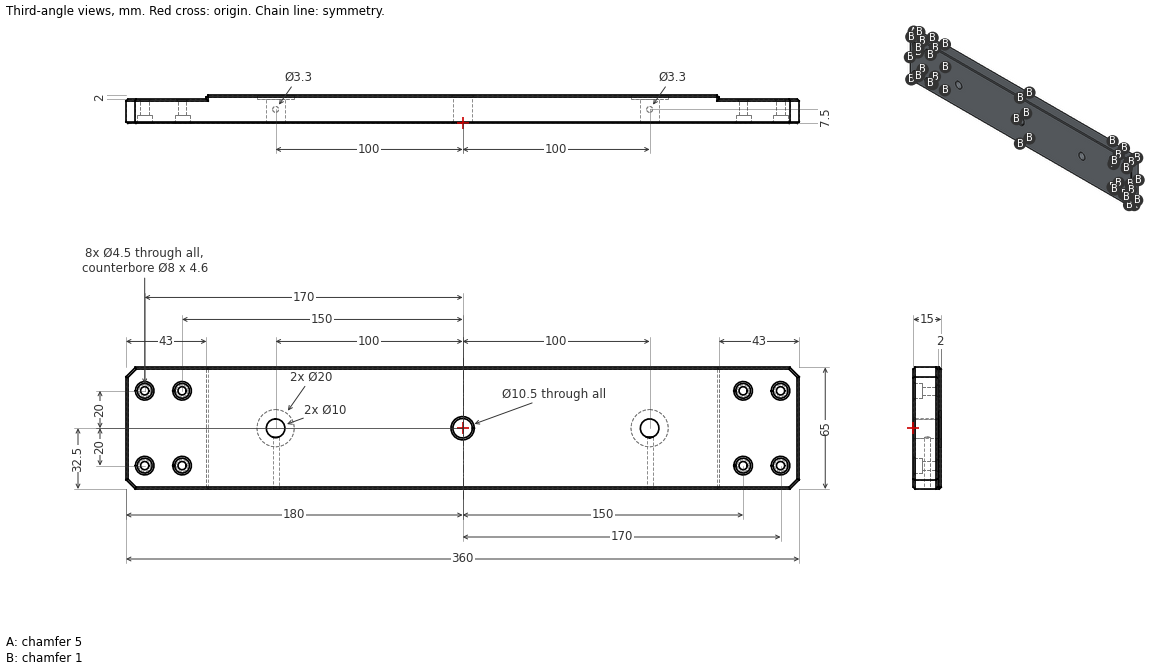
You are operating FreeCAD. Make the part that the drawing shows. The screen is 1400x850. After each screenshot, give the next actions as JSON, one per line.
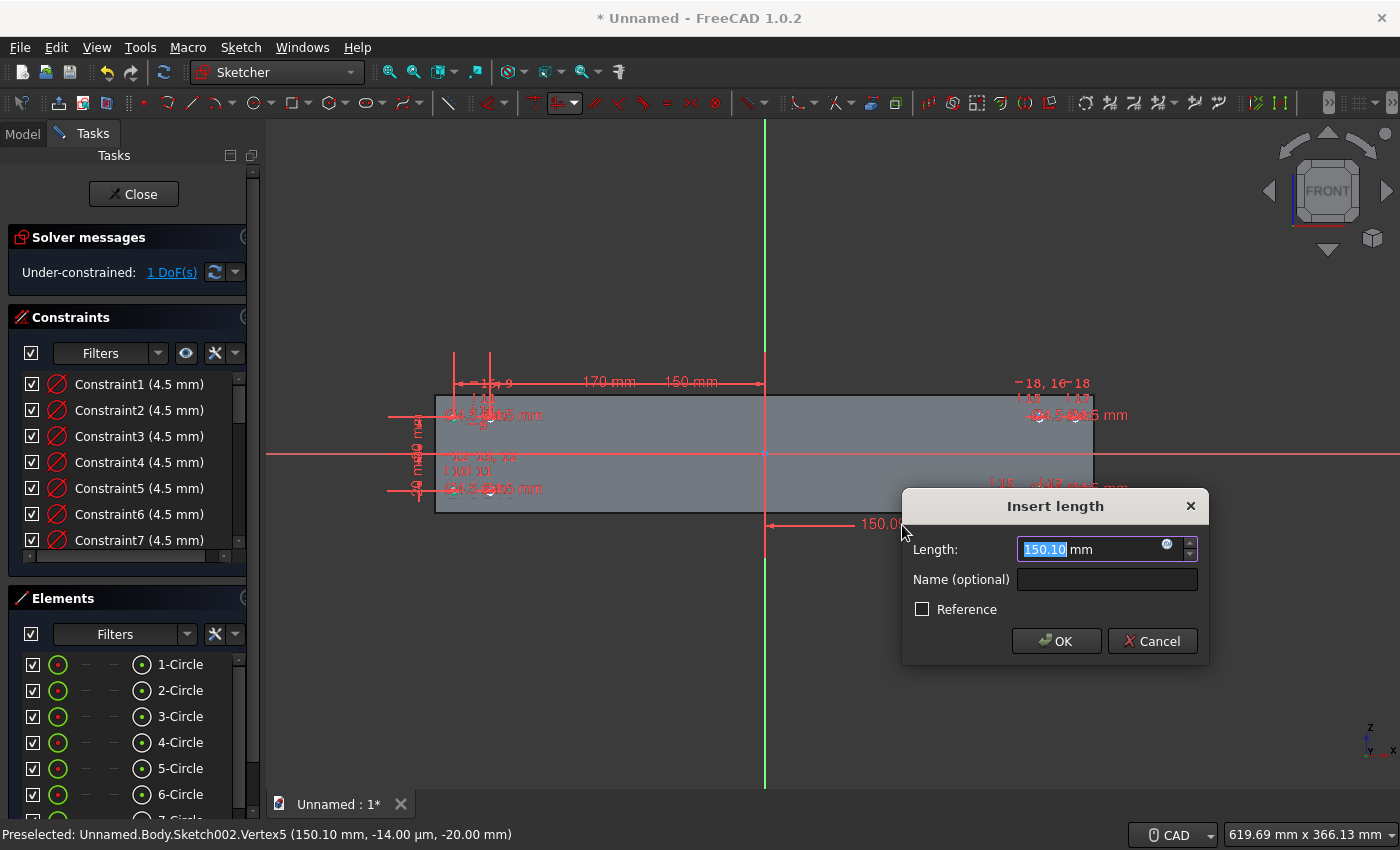
{"action": "type", "text": "150"}
{"action": "key", "text": "Return"}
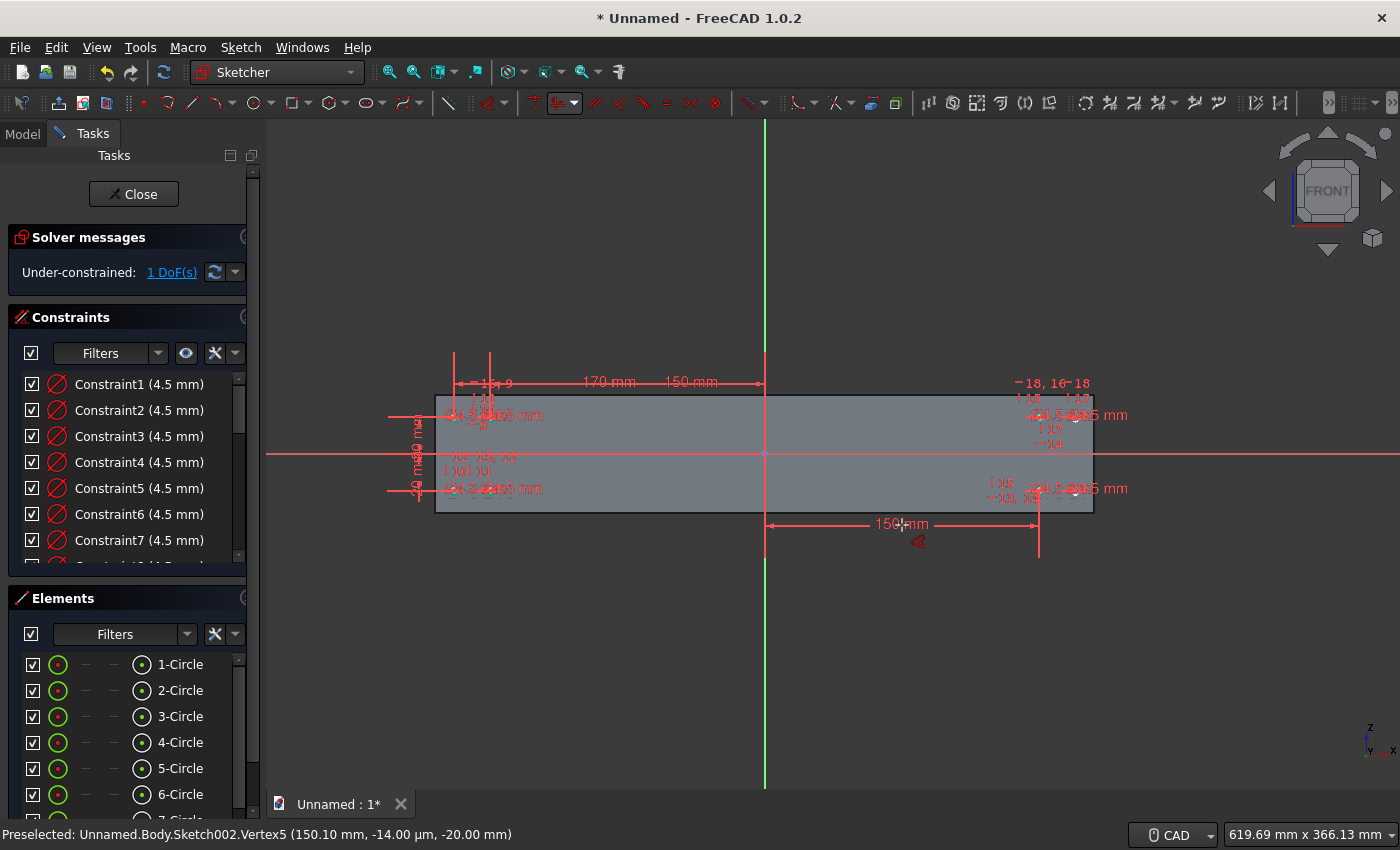
{"action": "left_click", "coordinate": [1075, 491]}
{"action": "left_click", "coordinate": [992, 525]}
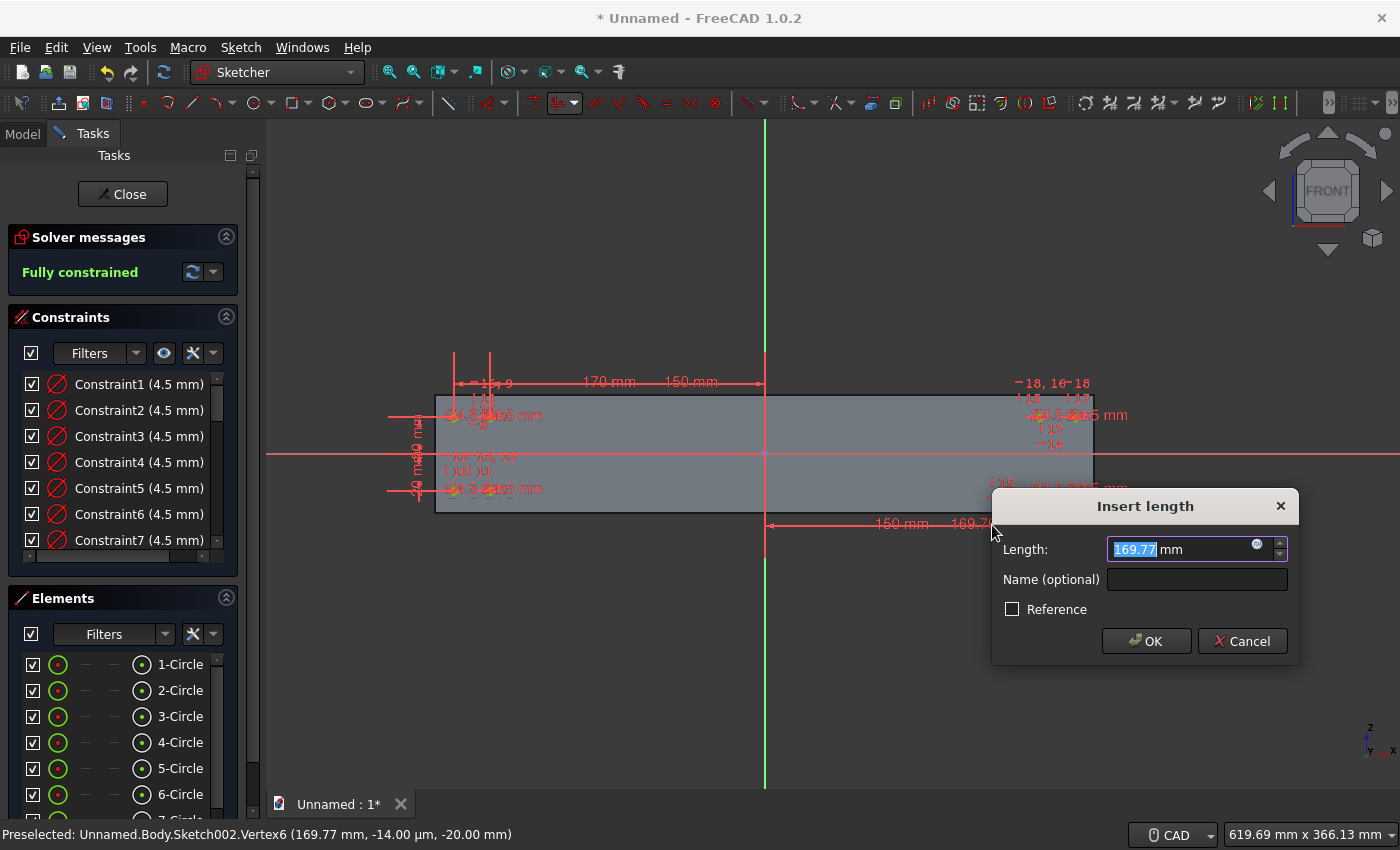
{"action": "type", "text": "170"}
{"action": "key", "text": "Return"}
{"action": "key", "text": "Escape"}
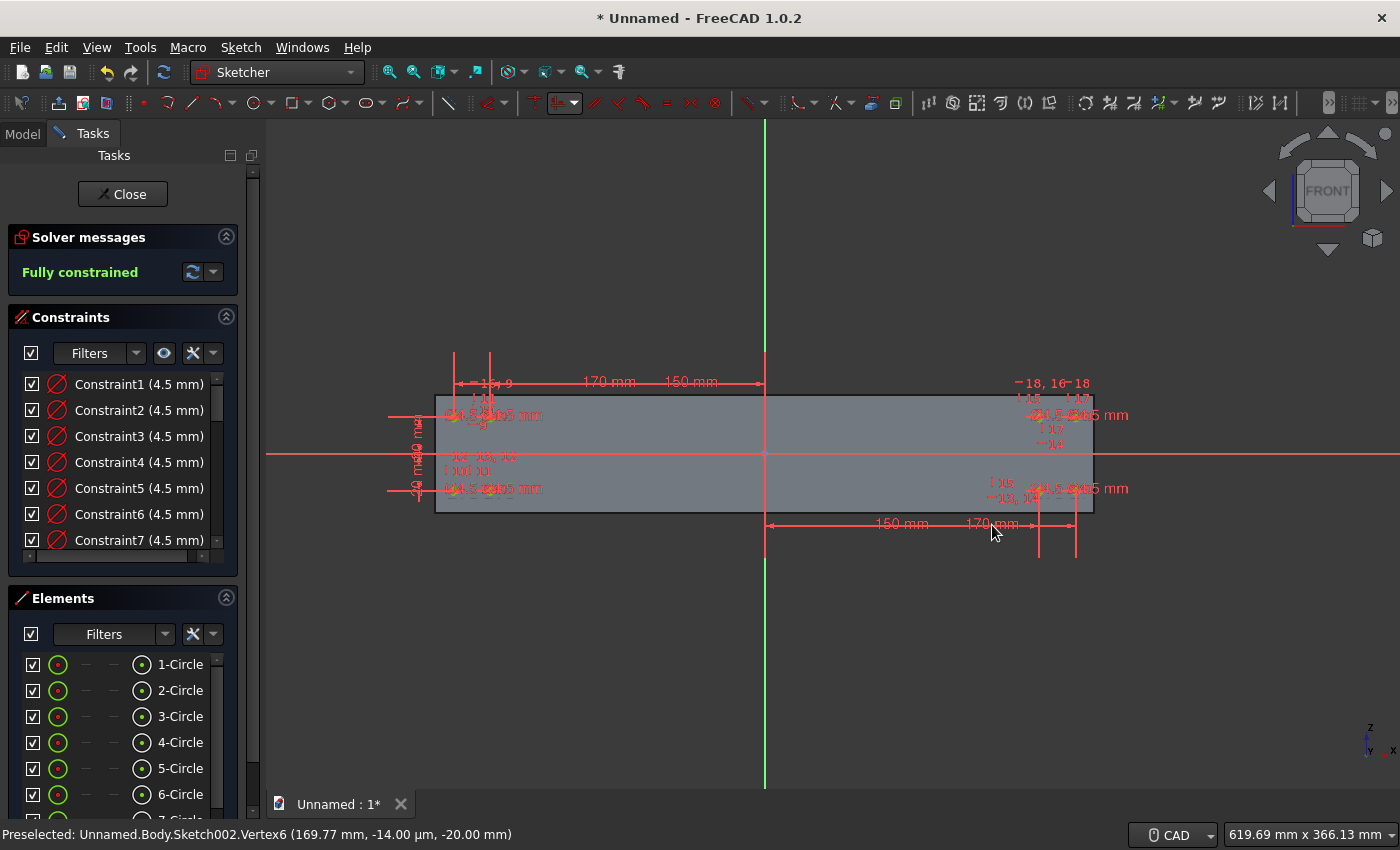
{"action": "left_click", "coordinate": [123, 194]}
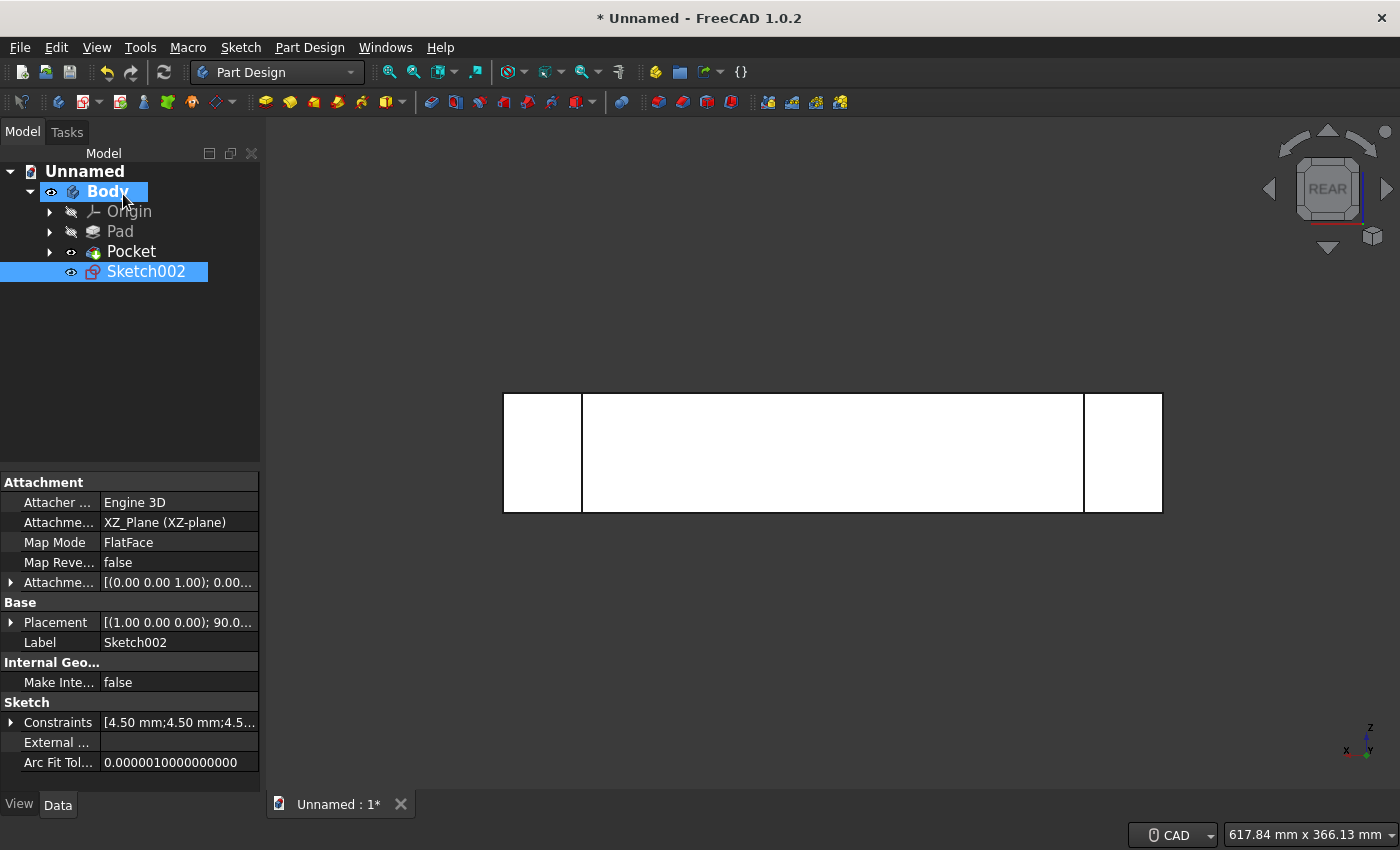
{"action": "left_click", "coordinate": [456, 102]}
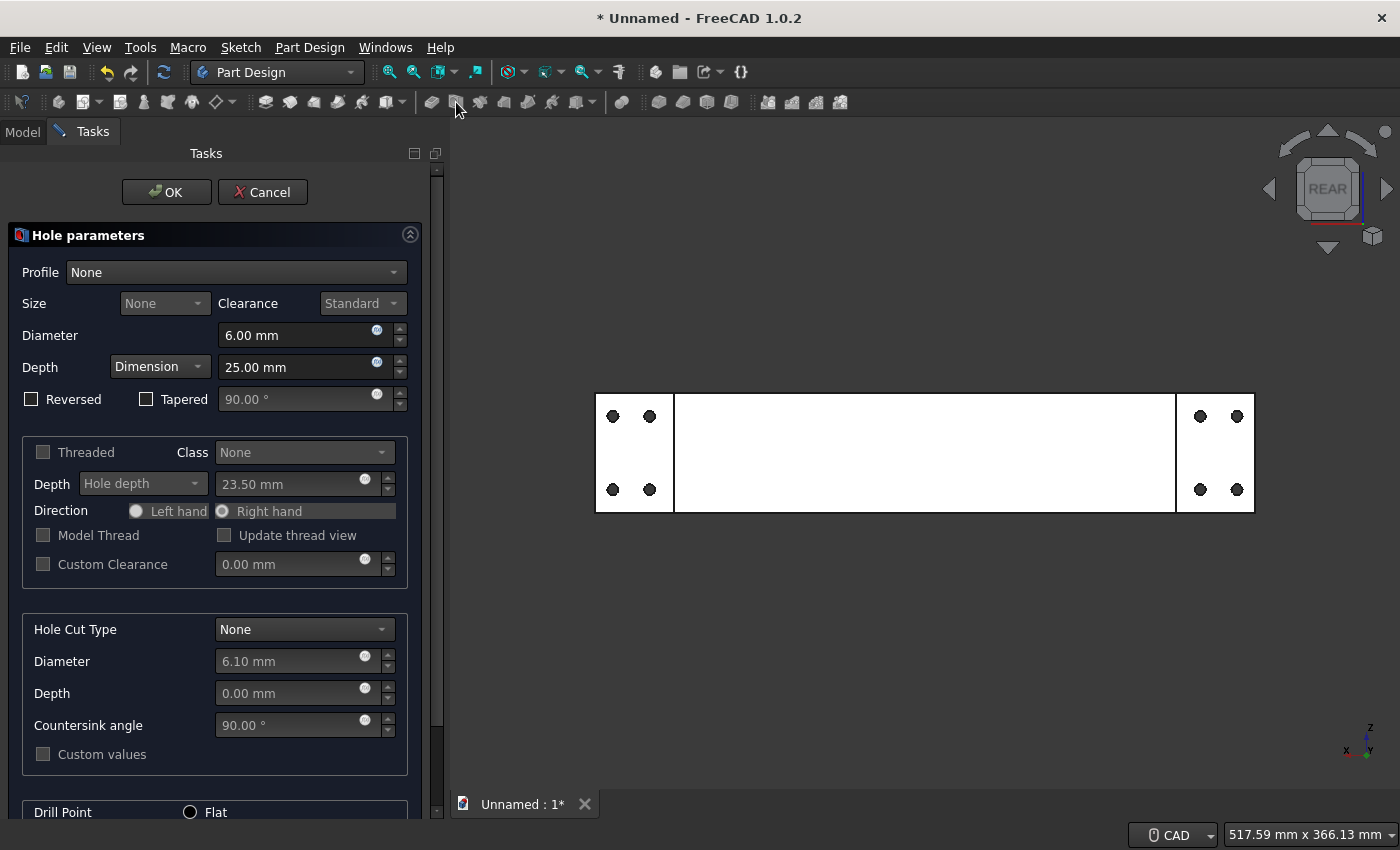
{"action": "triple_click", "coordinate": [305, 335]}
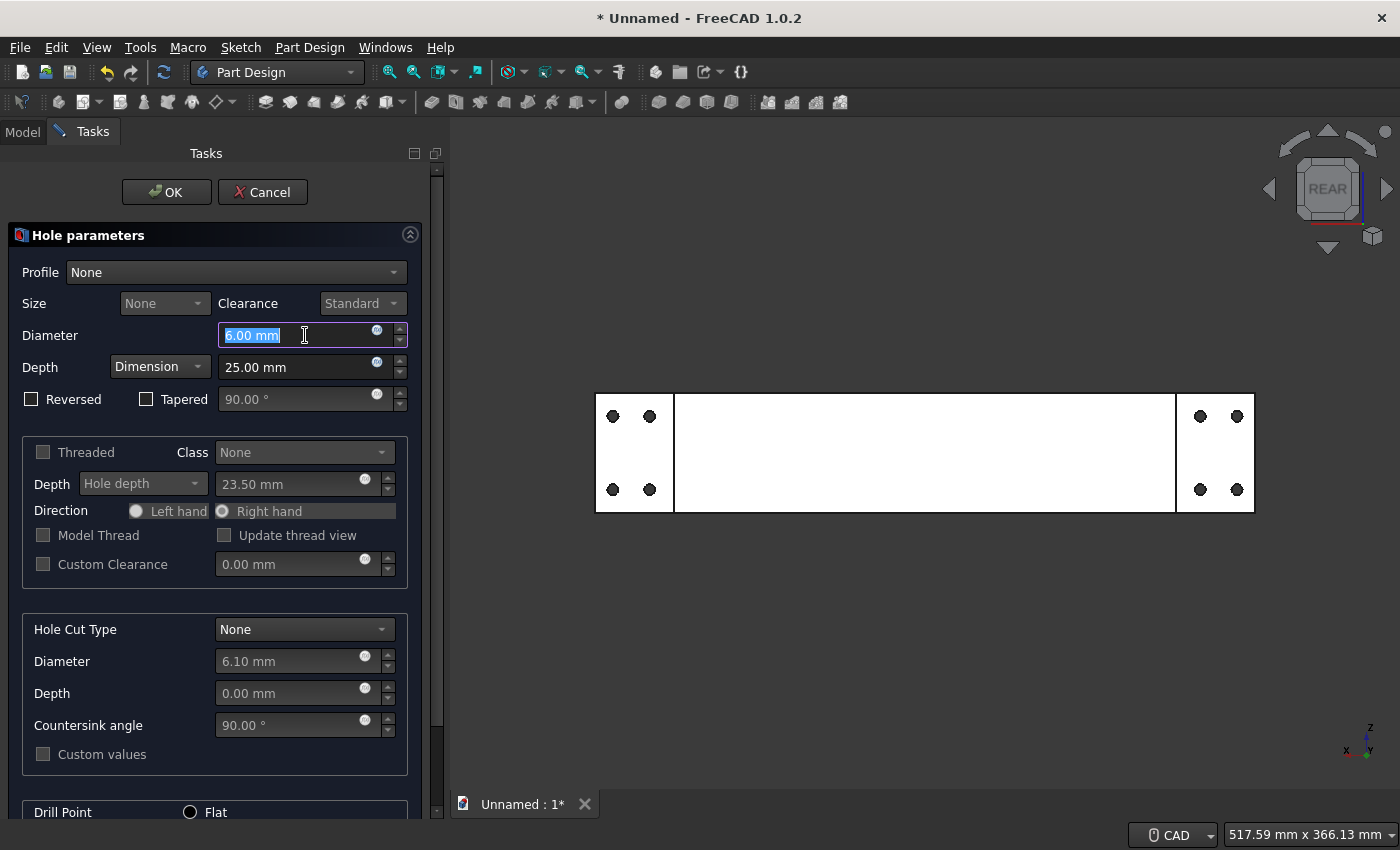
{"action": "type", "text": "4.5"}
{"action": "key", "text": "Tab"}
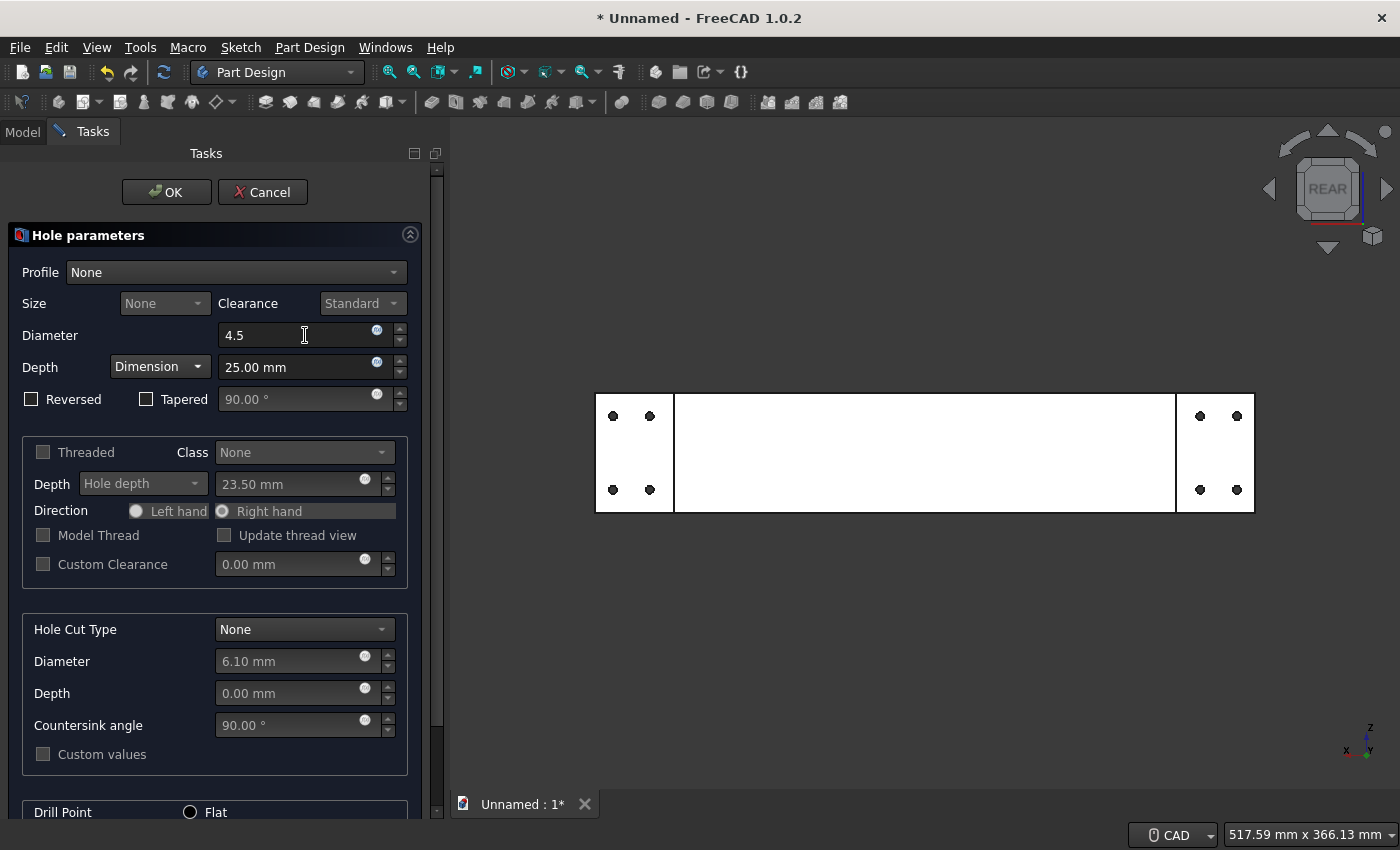
{"action": "left_click", "coordinate": [161, 366]}